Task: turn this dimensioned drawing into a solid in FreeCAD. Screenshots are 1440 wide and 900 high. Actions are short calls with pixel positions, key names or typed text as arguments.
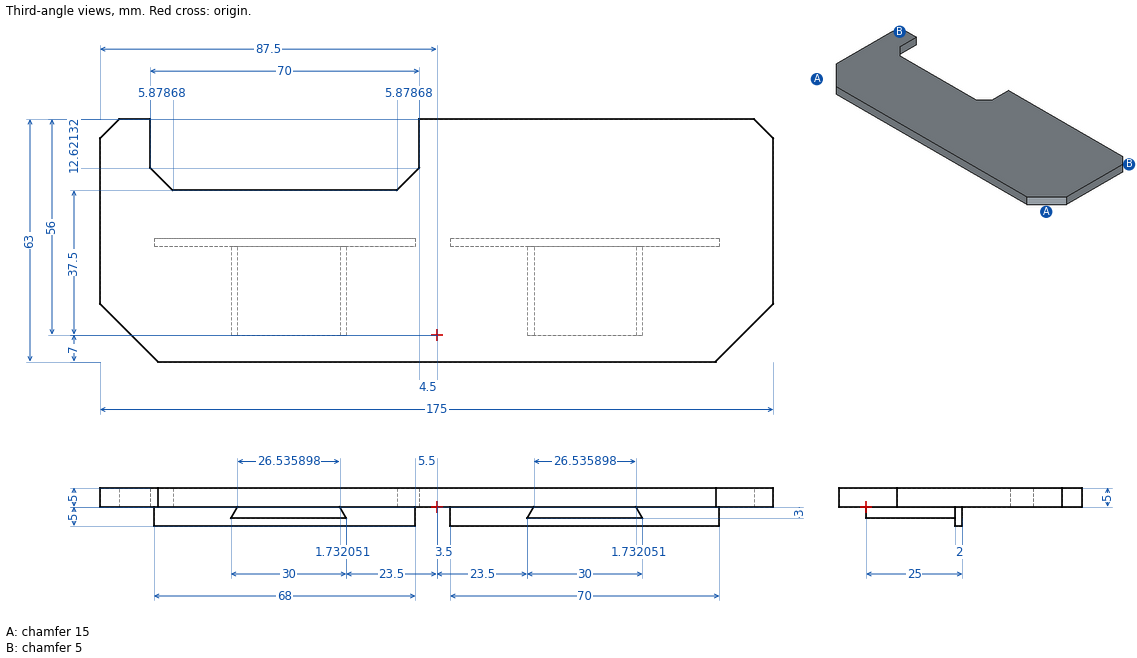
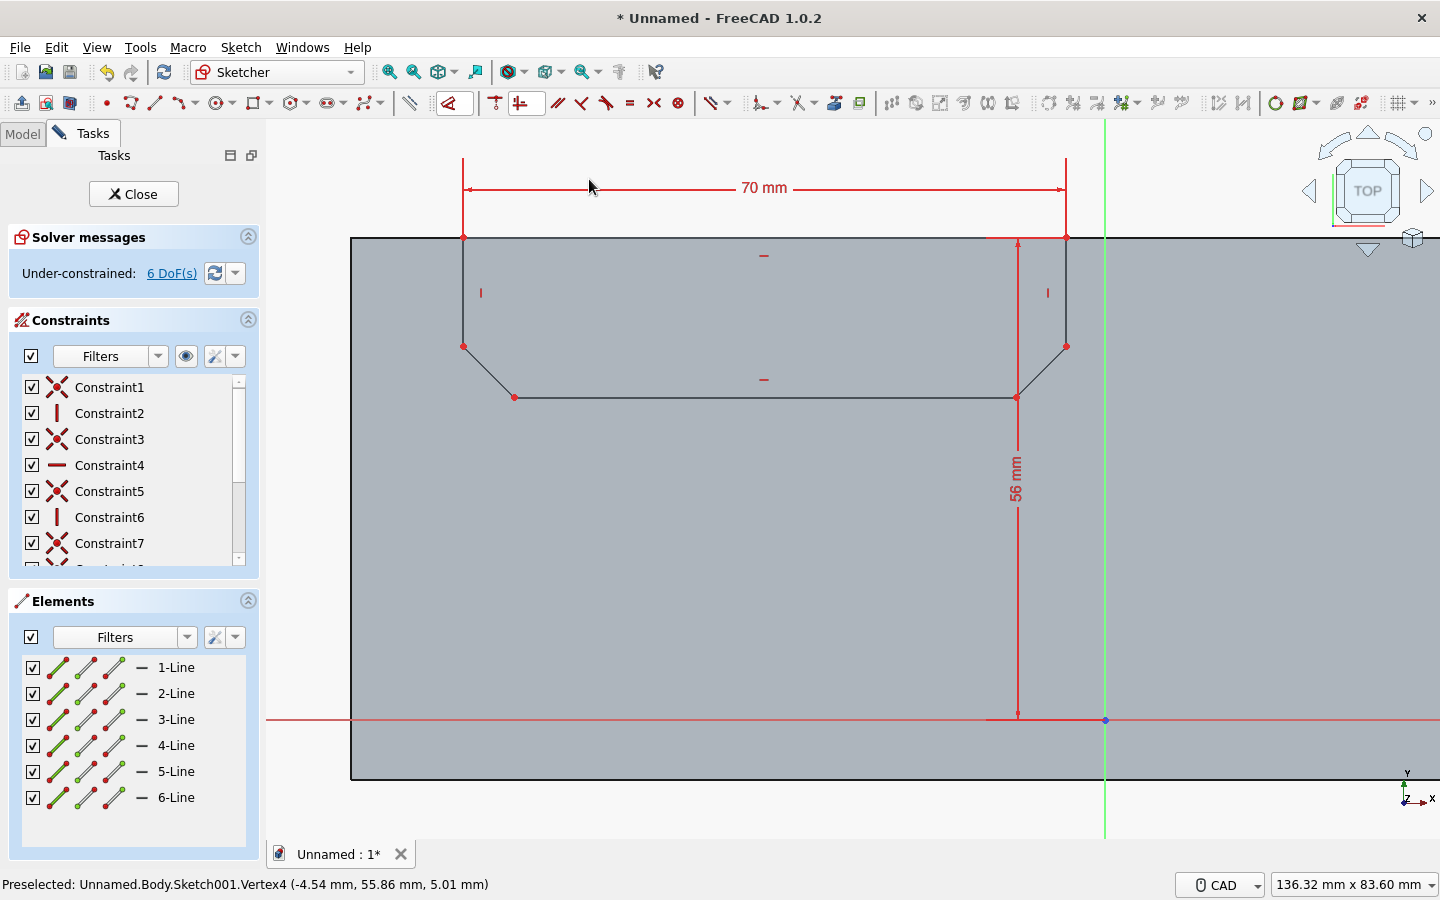
click(1066, 347)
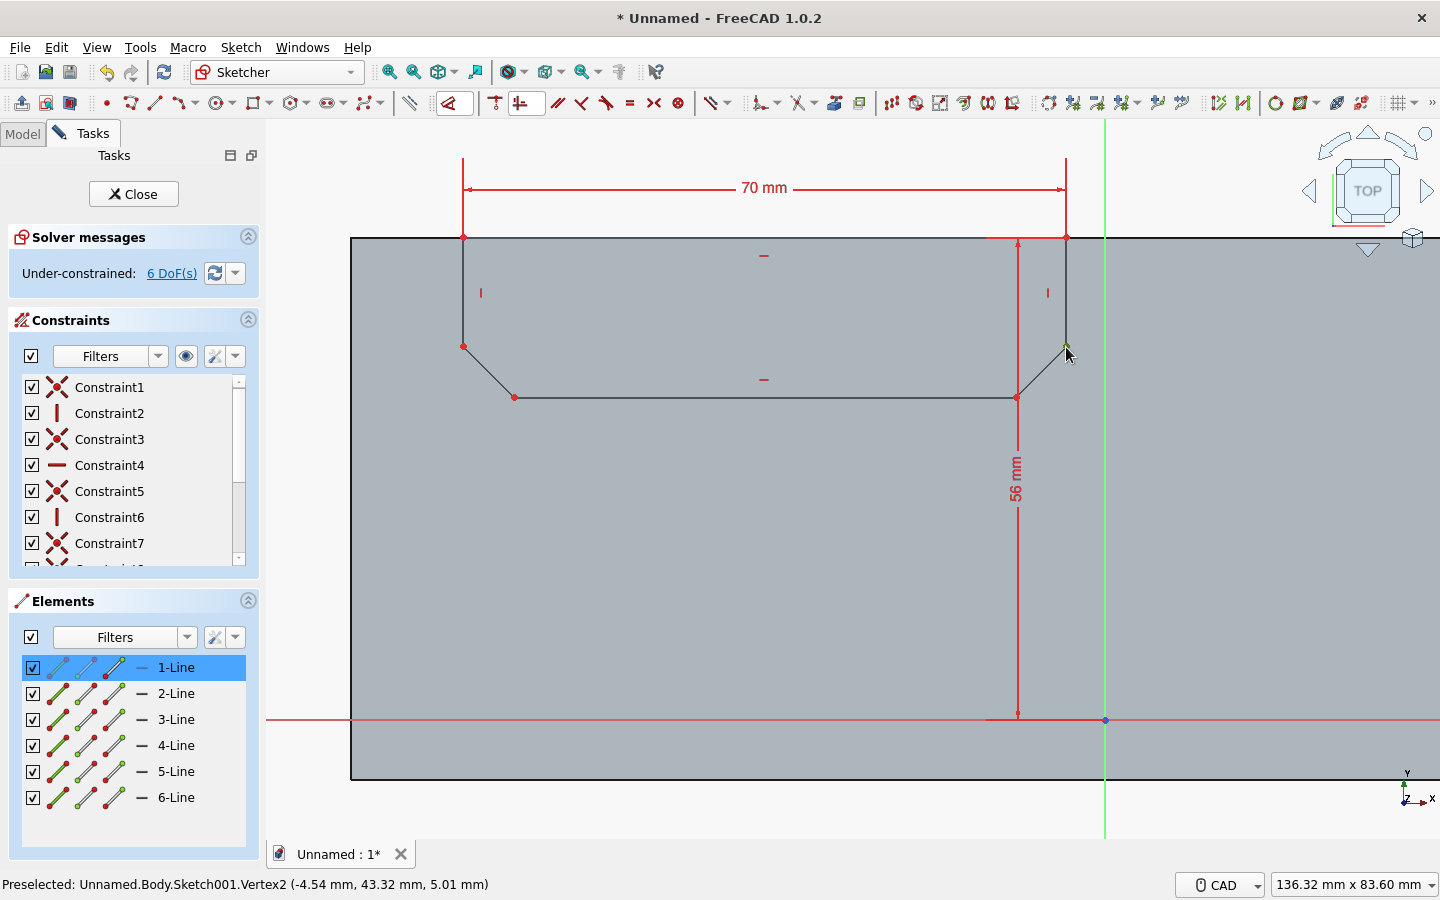
click(468, 104)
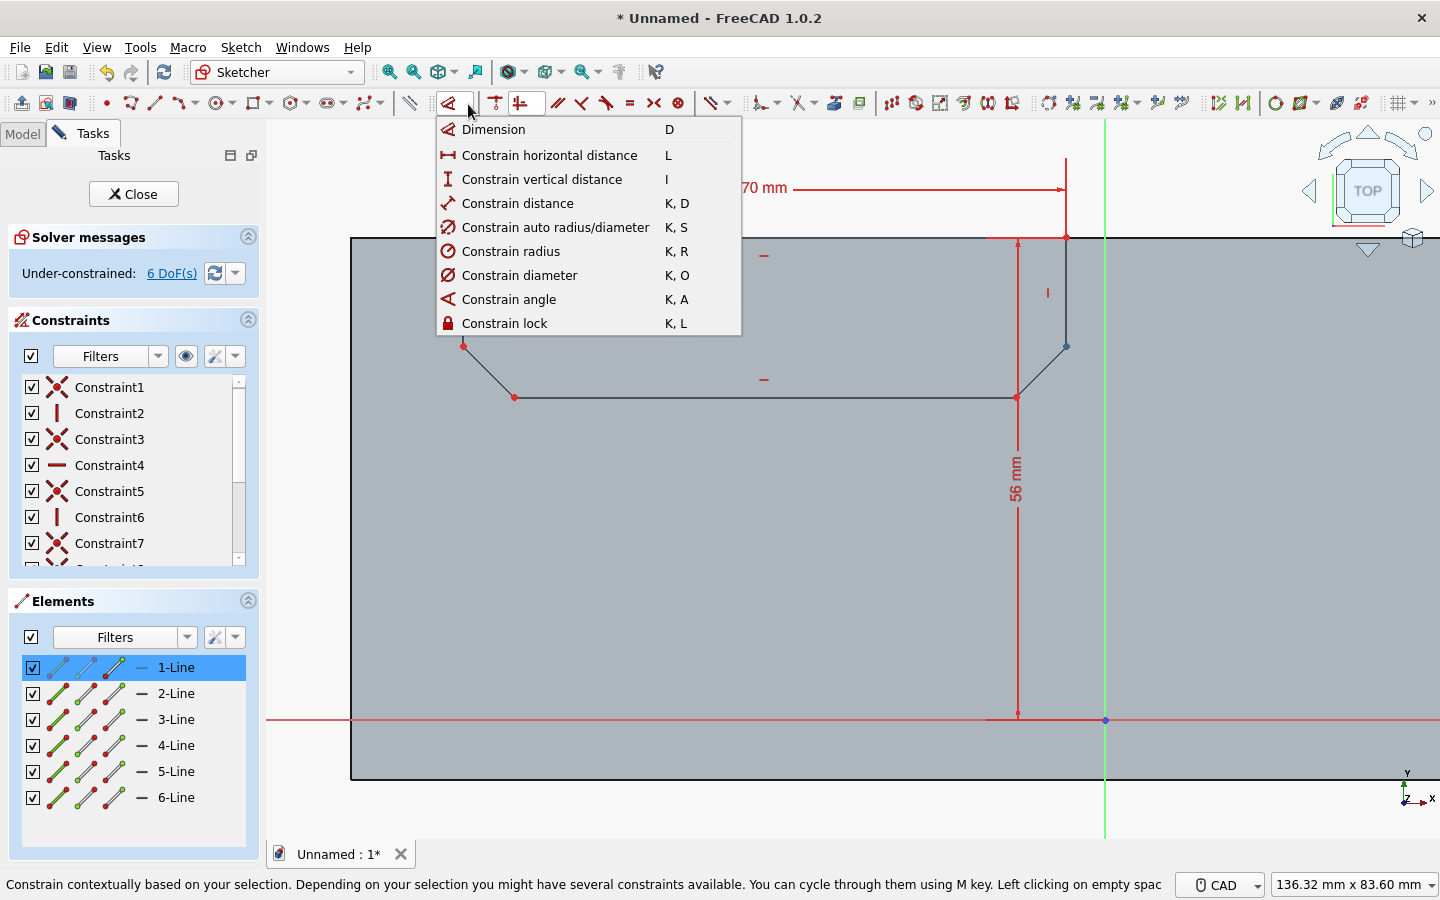
click(589, 155)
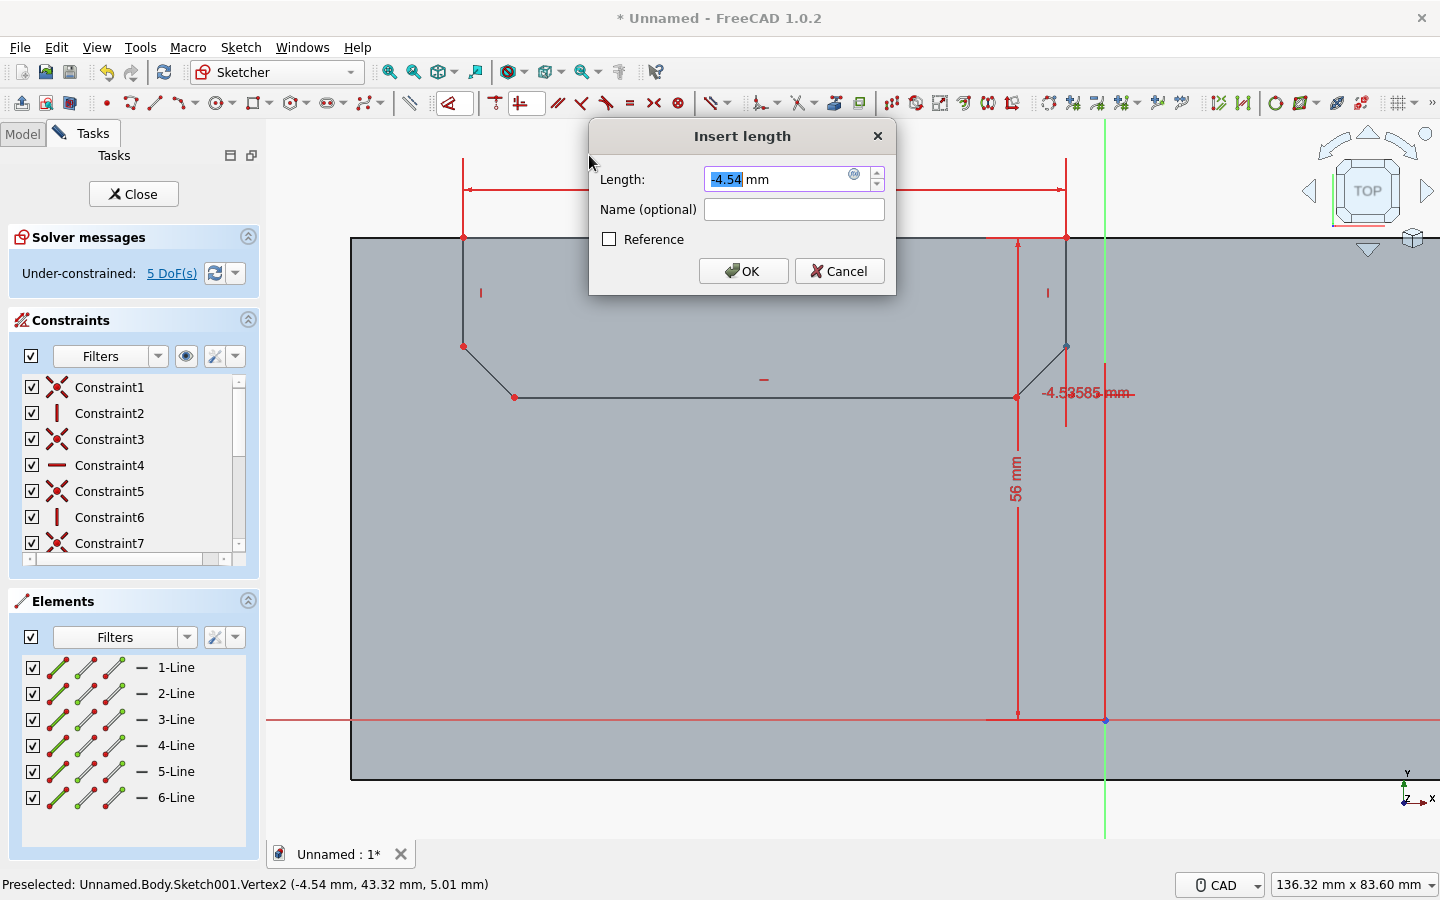
text(-4.5)
key(Return)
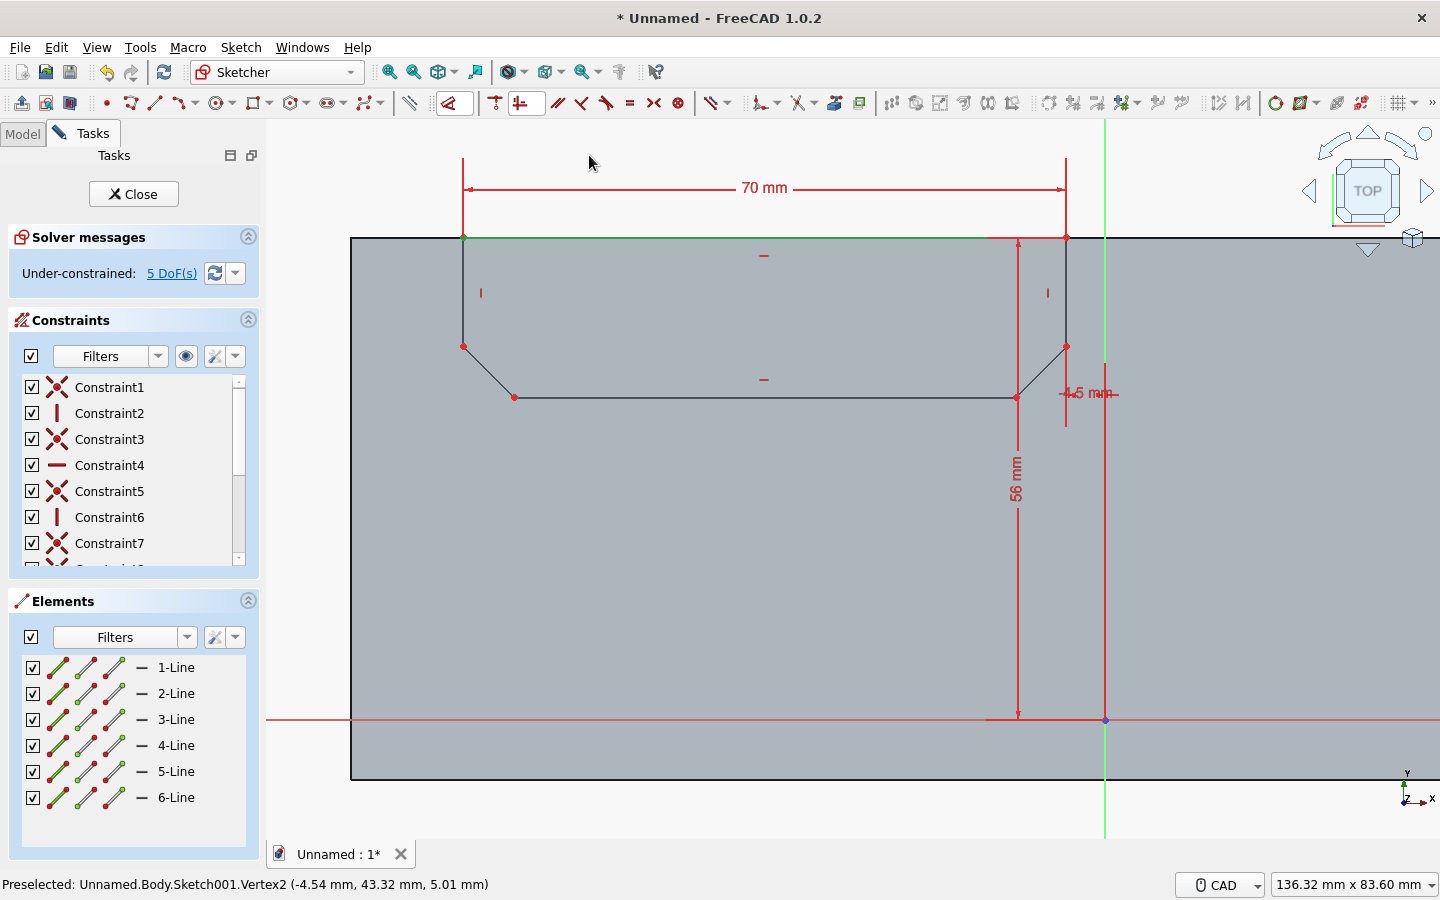
click(1016, 398)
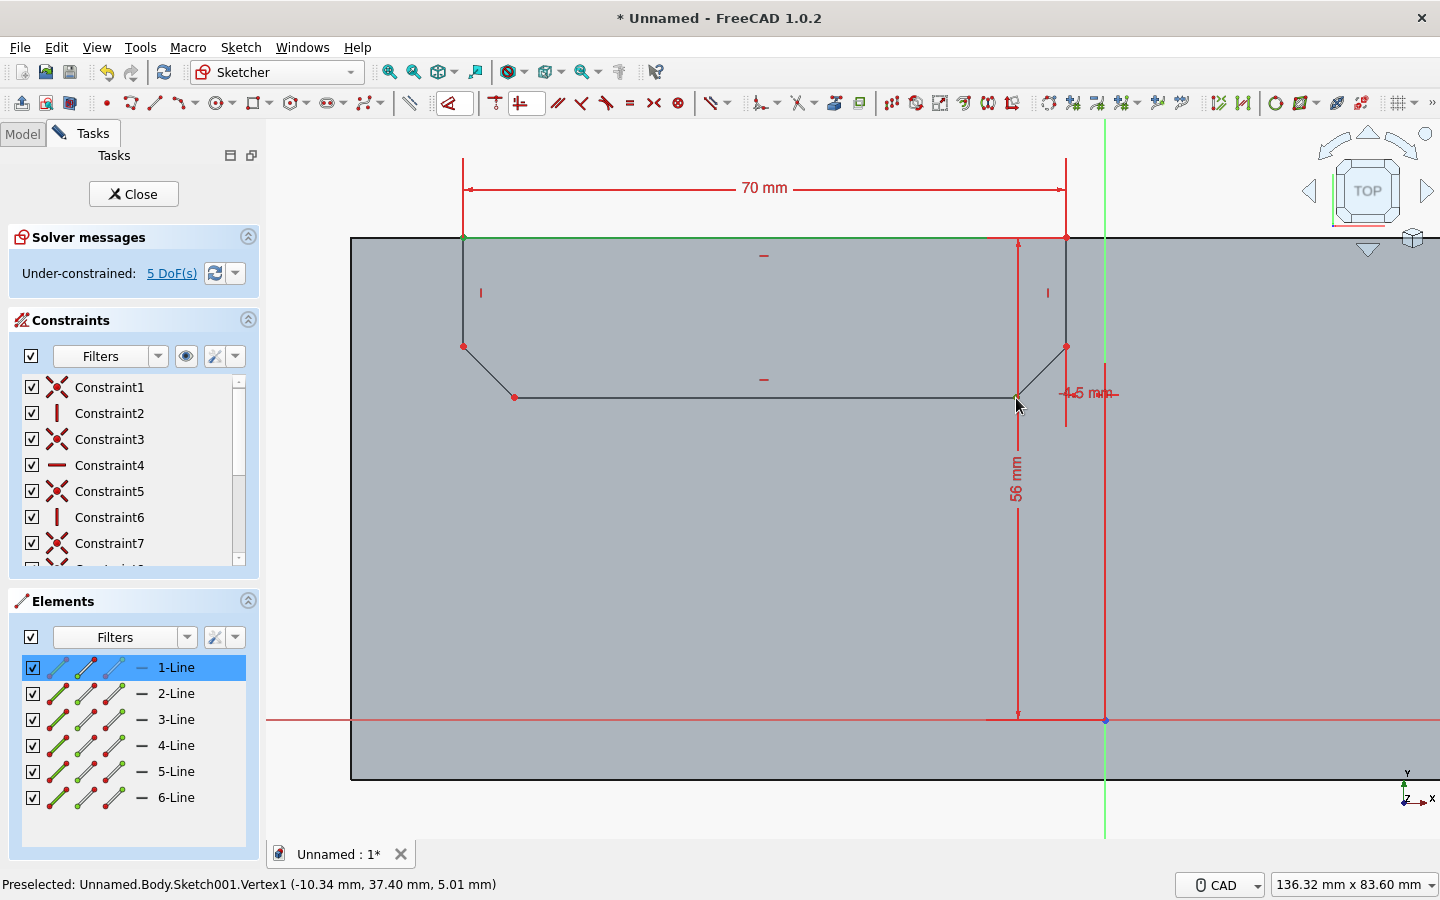
key(i)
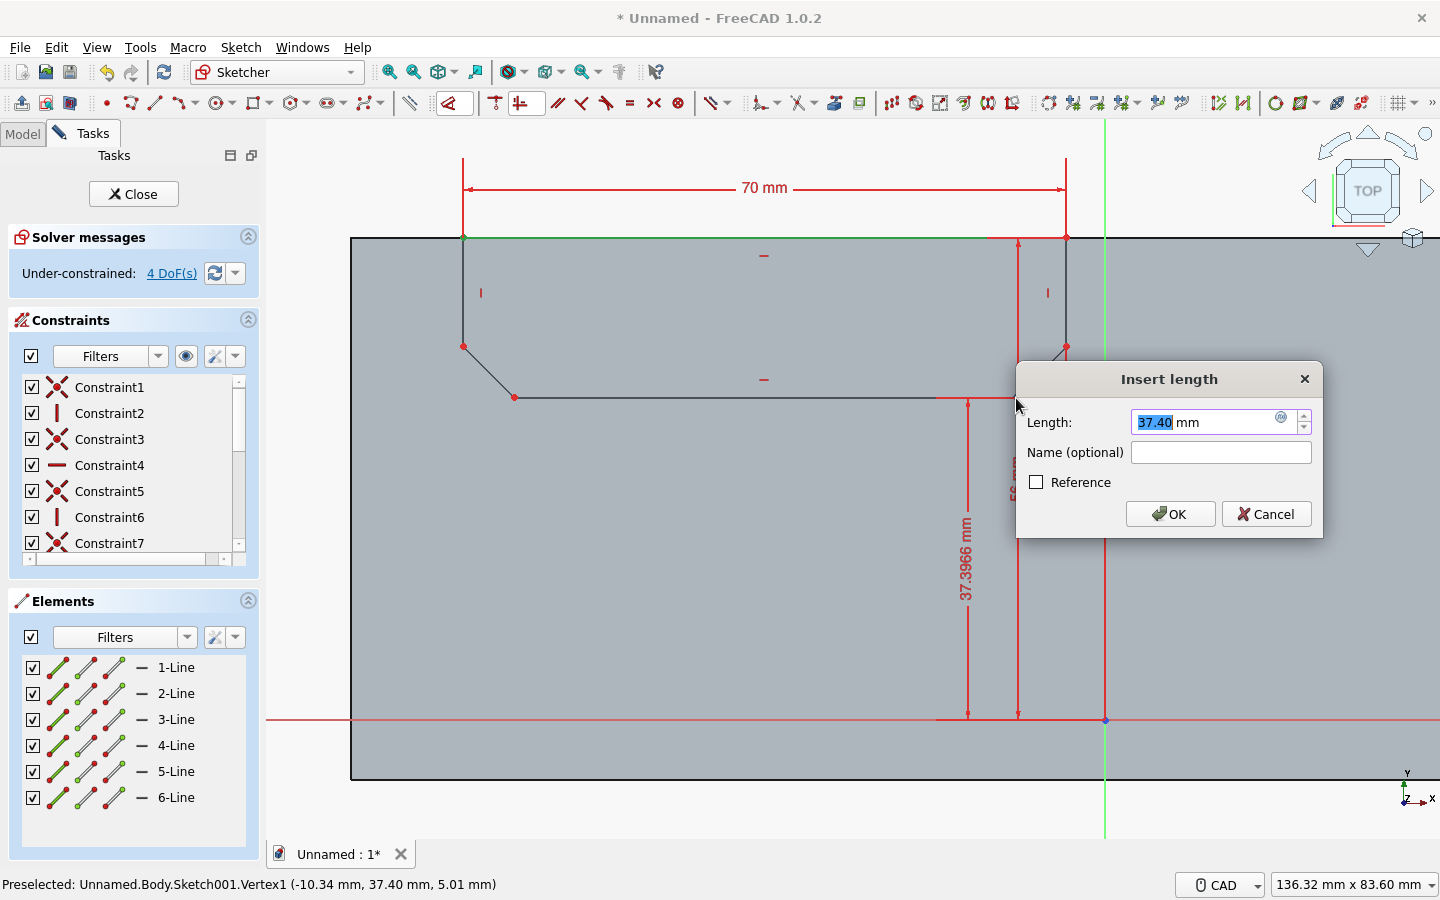
text(37.5)
key(Return)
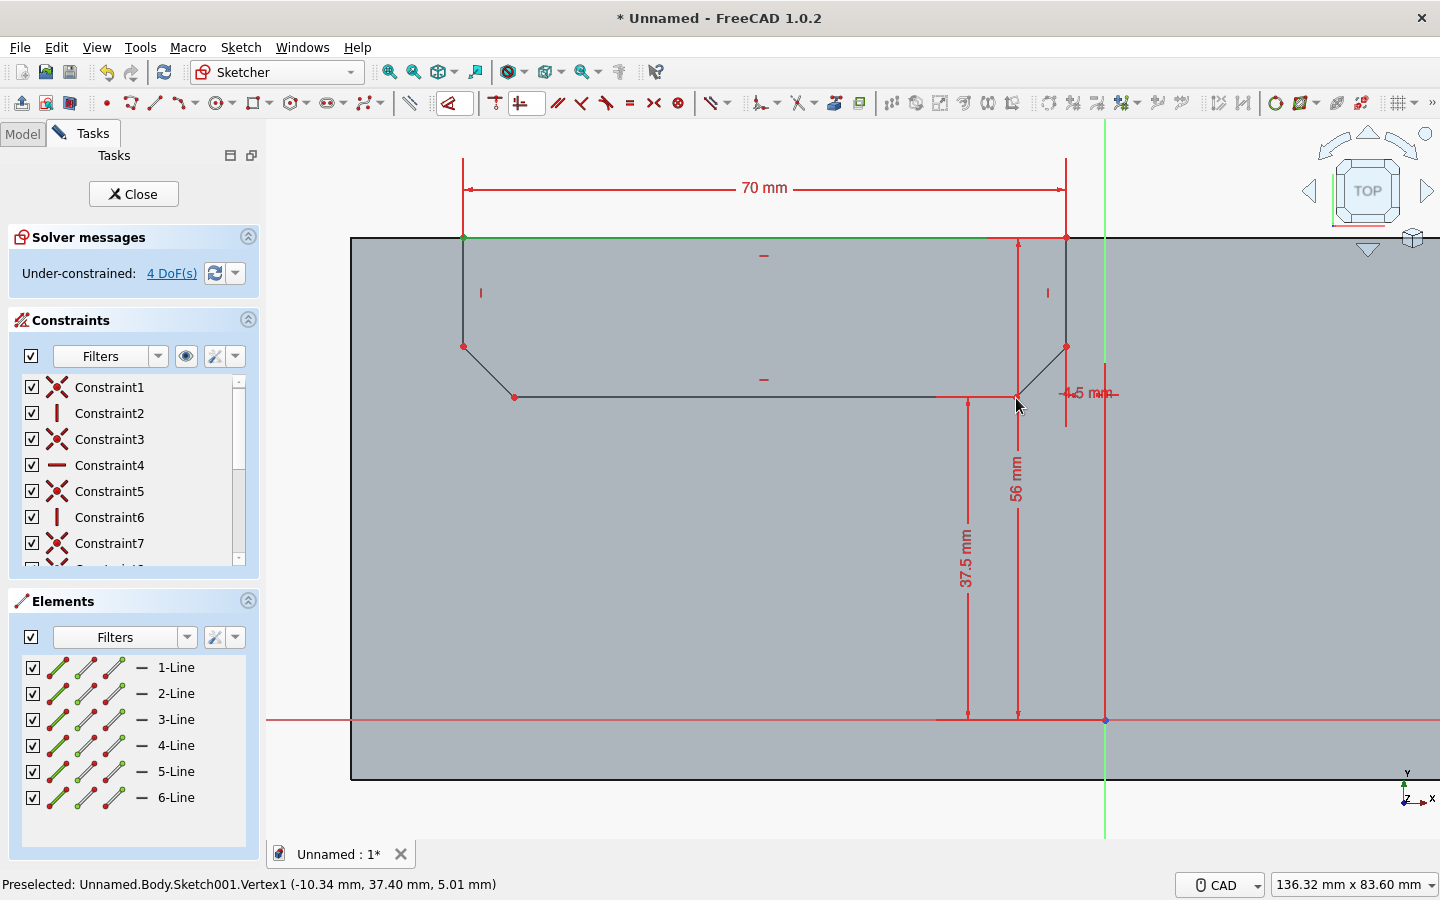
click(1066, 314)